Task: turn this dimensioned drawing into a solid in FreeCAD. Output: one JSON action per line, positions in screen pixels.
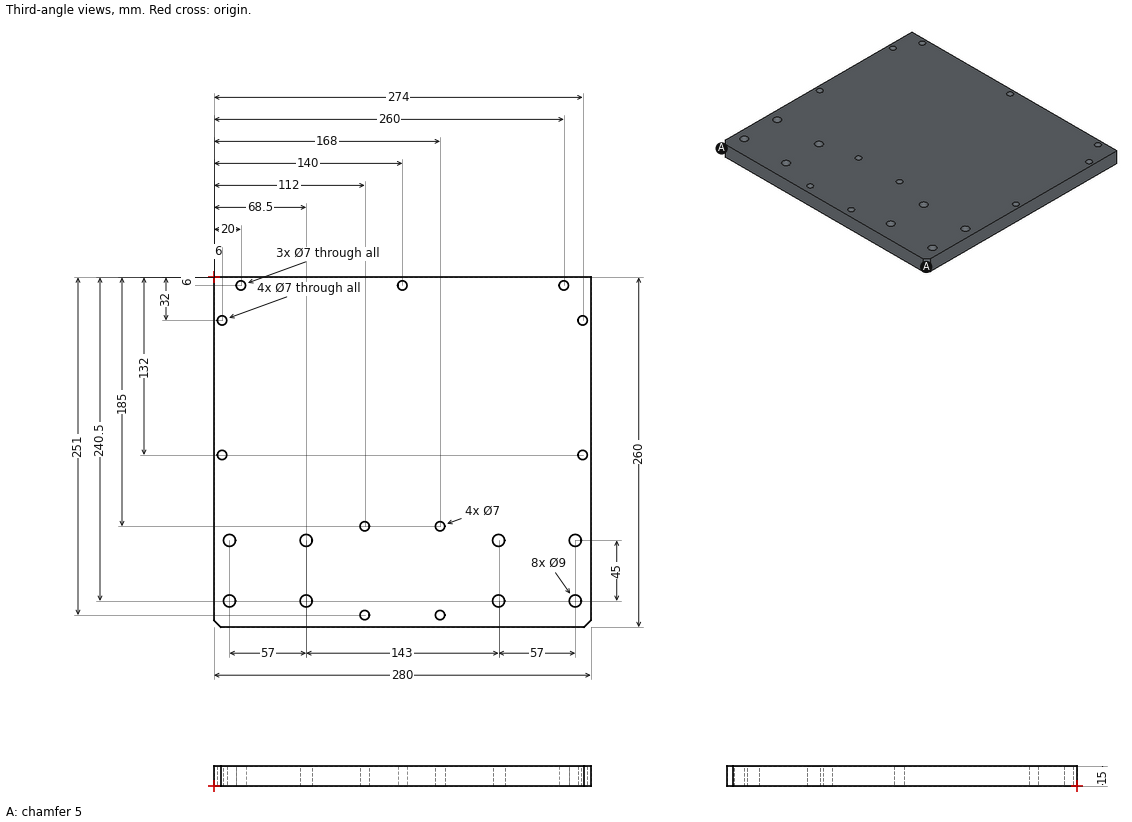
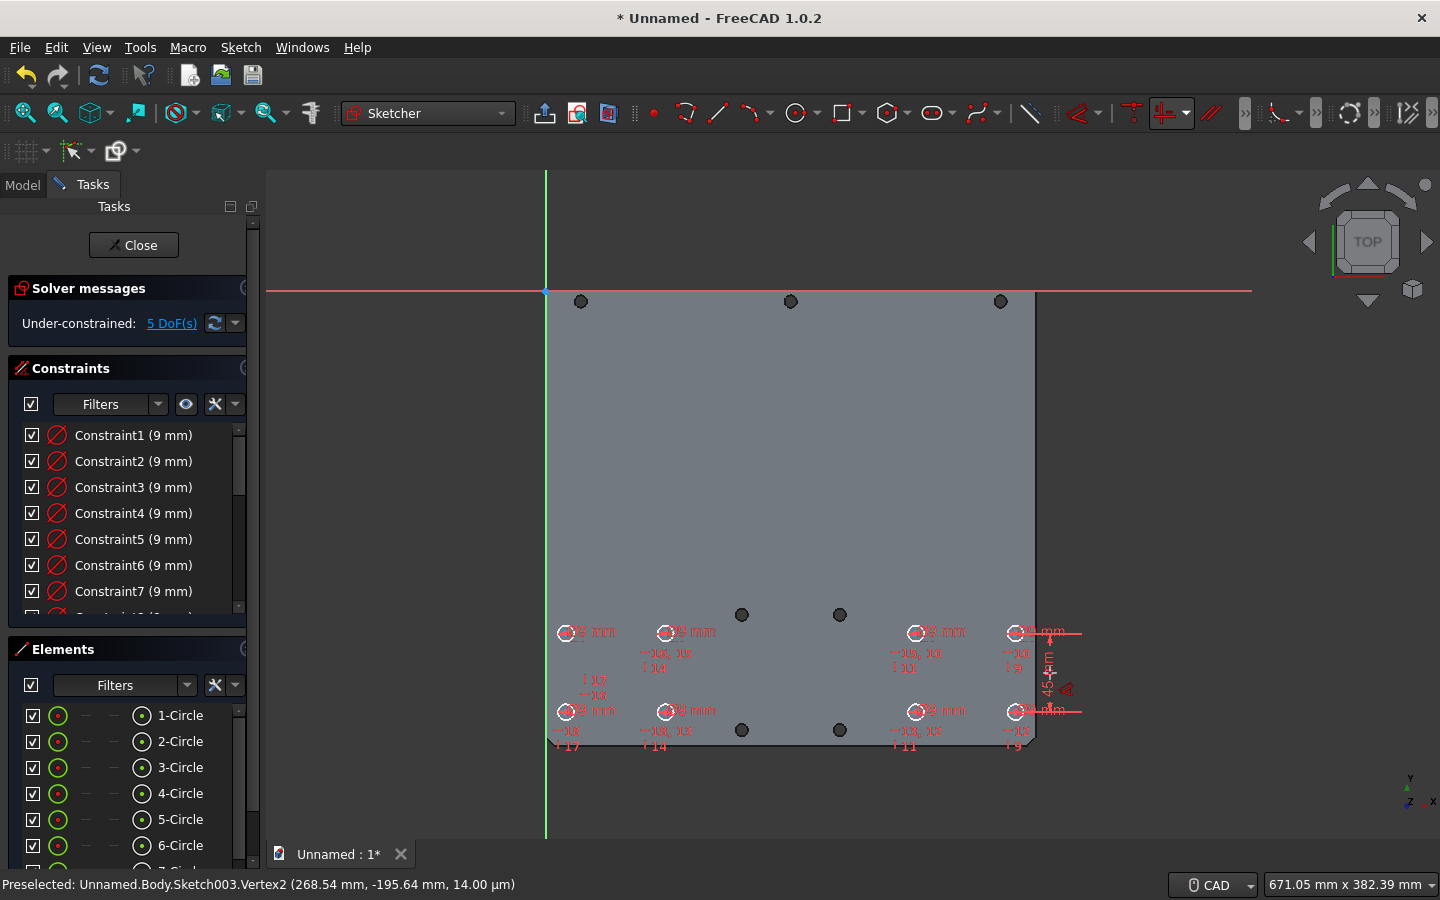
{"action": "left_click", "coordinate": [1016, 634]}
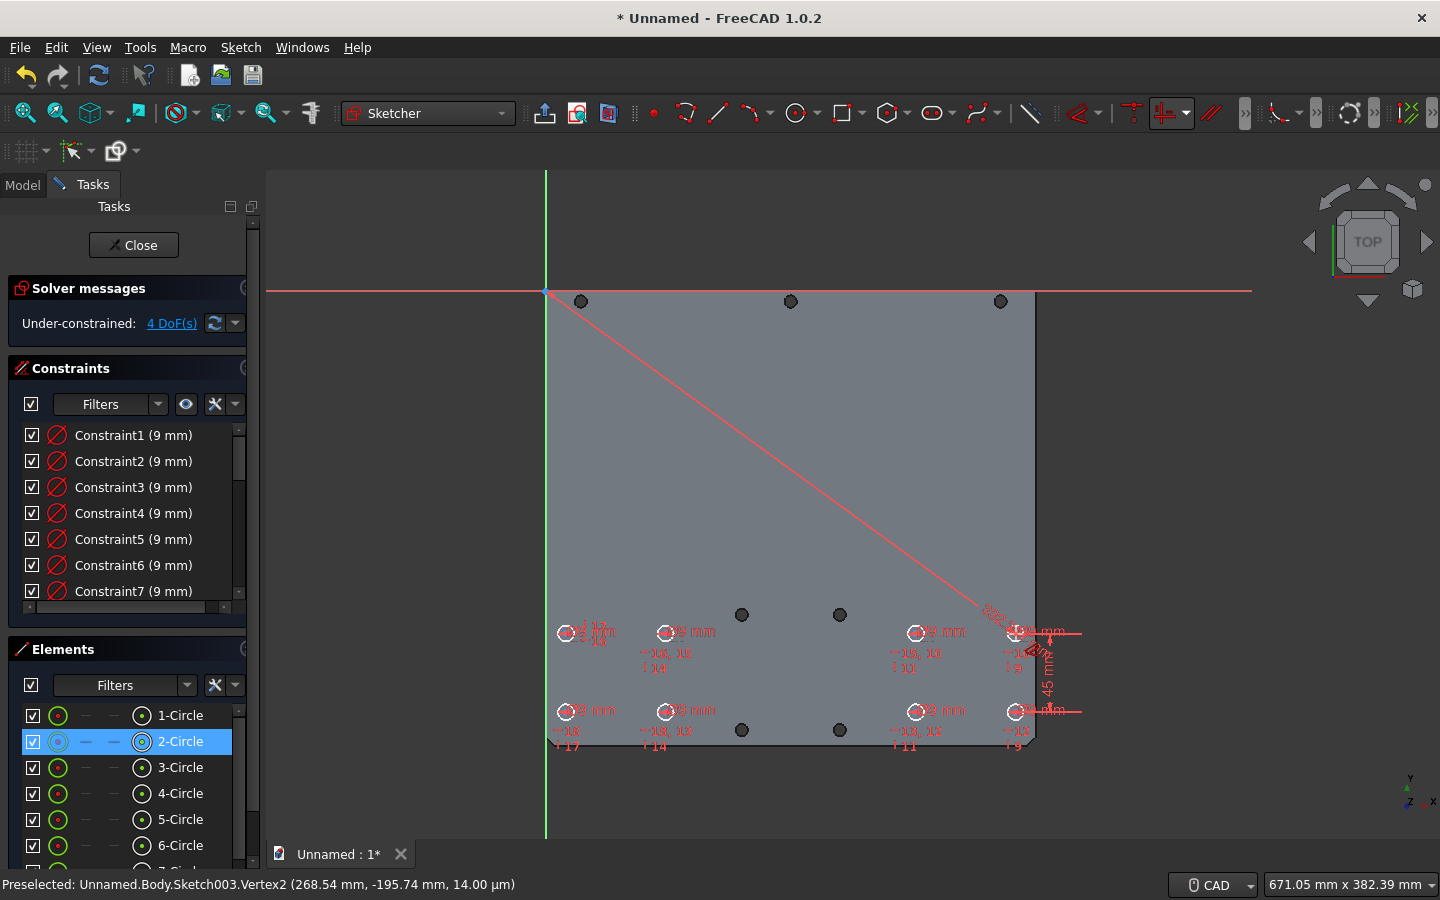
{"action": "left_click", "coordinate": [916, 634]}
{"action": "left_click", "coordinate": [966, 668]}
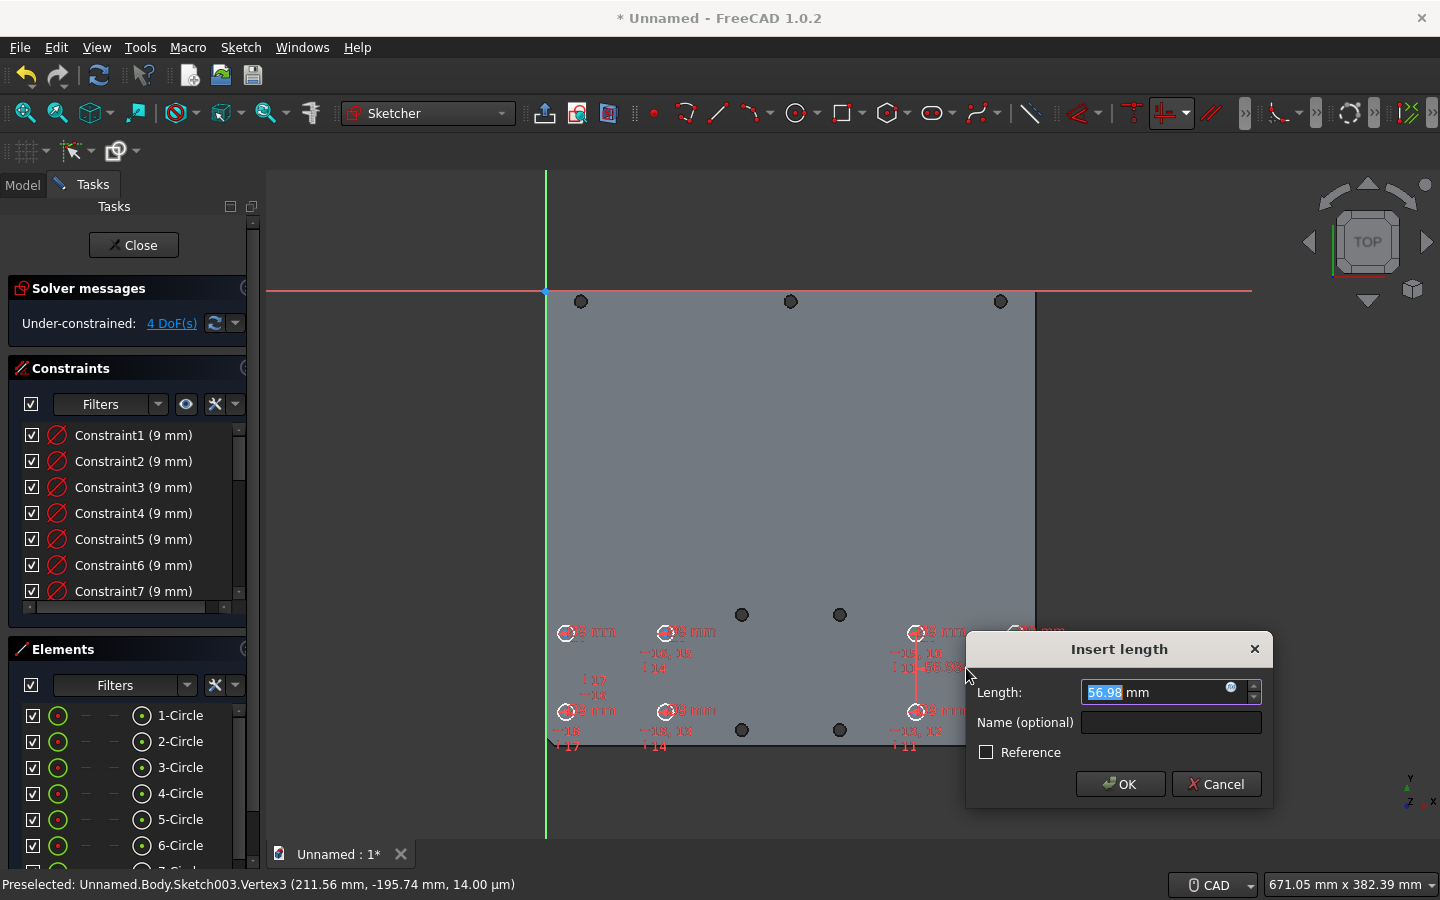
{"action": "type", "text": "57"}
{"action": "key", "text": "Return"}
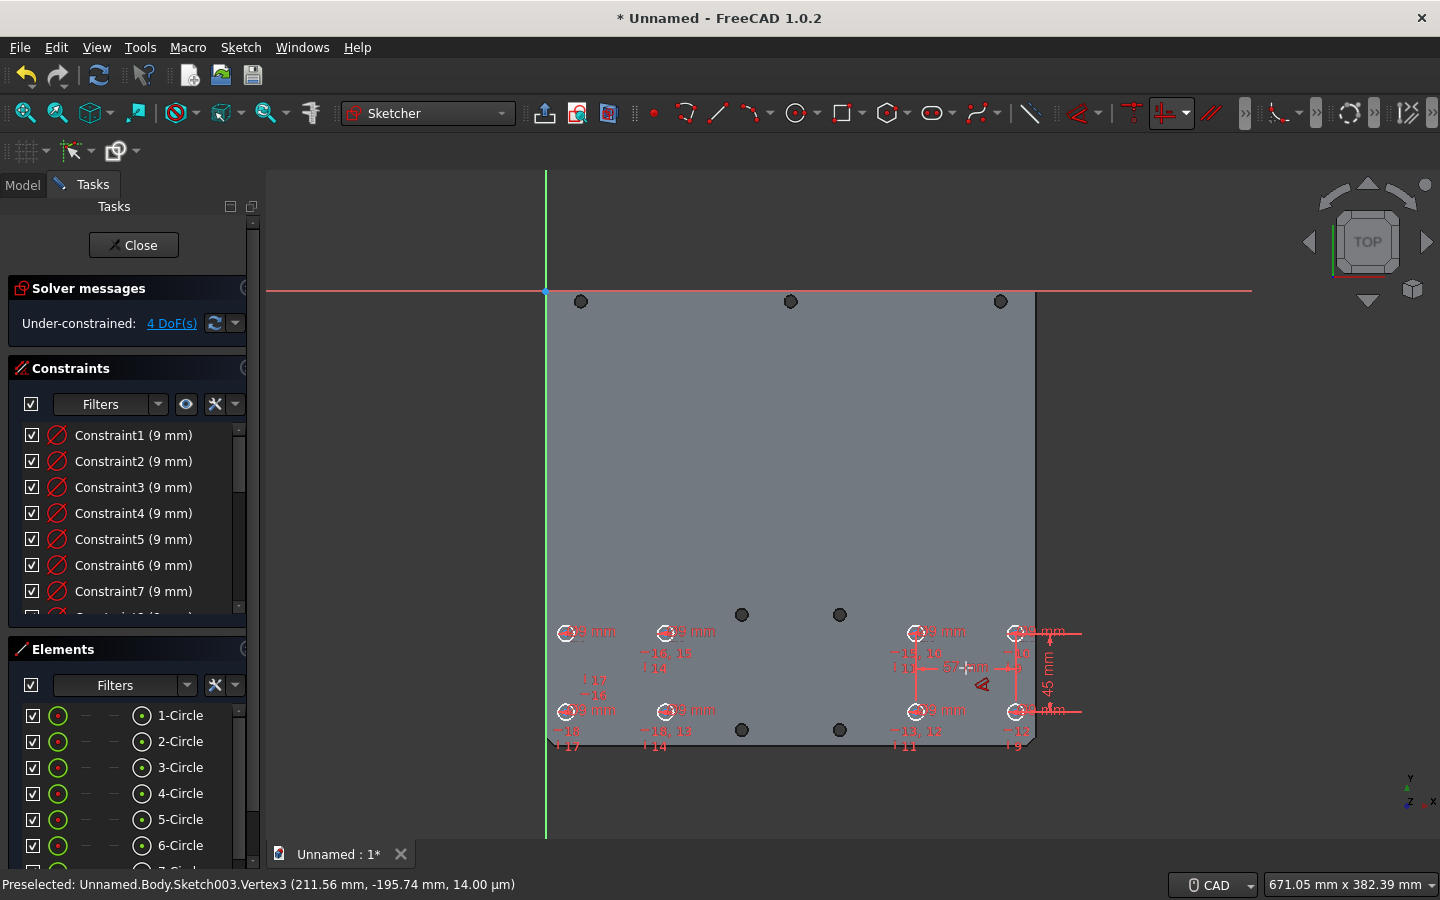
{"action": "left_click", "coordinate": [666, 634]}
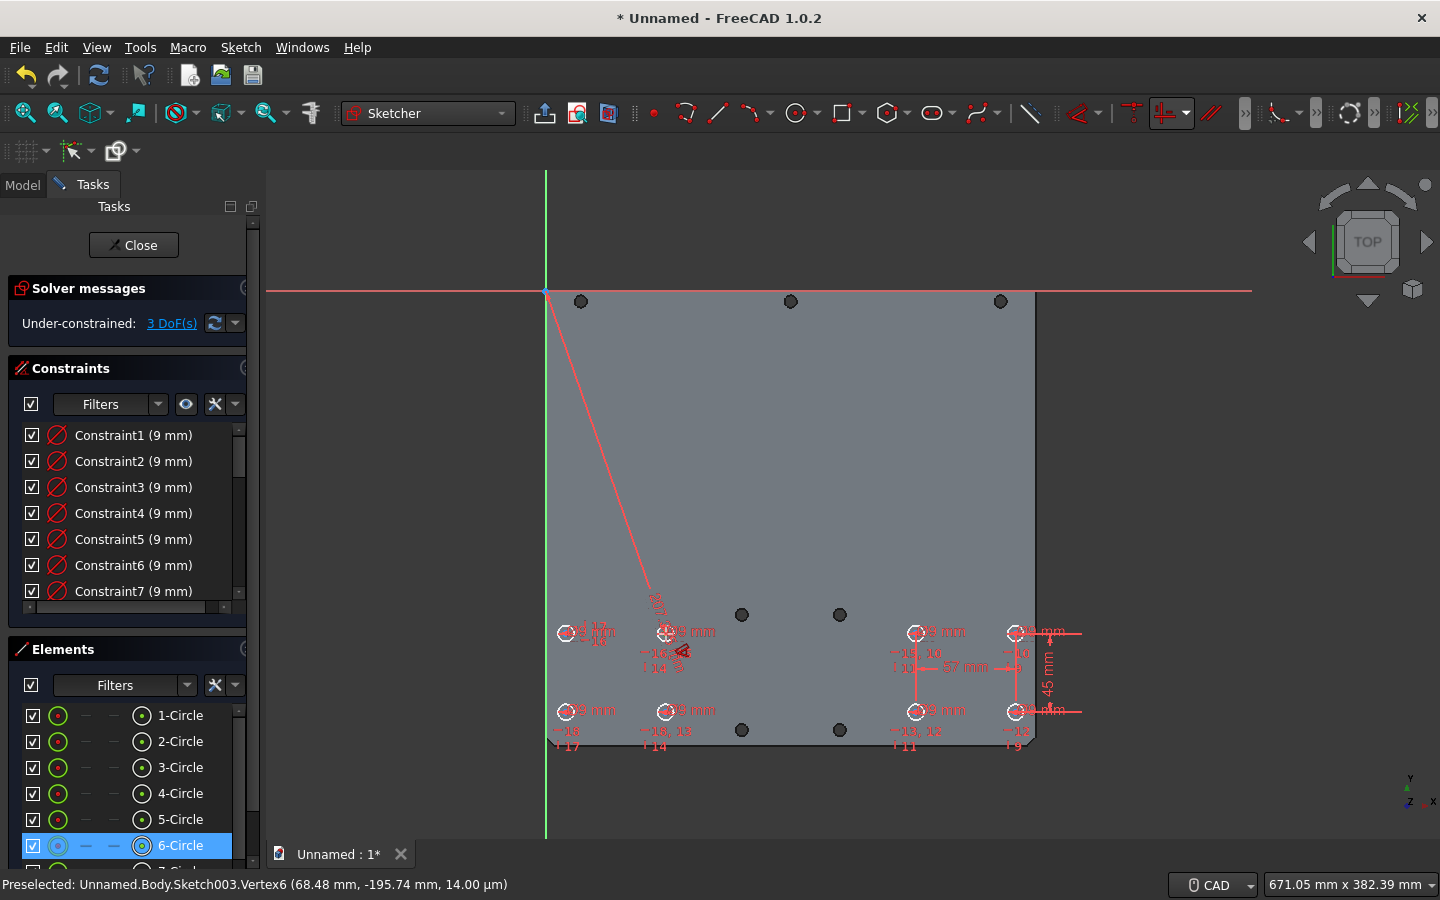
{"action": "left_click", "coordinate": [566, 634]}
{"action": "left_click", "coordinate": [616, 668]}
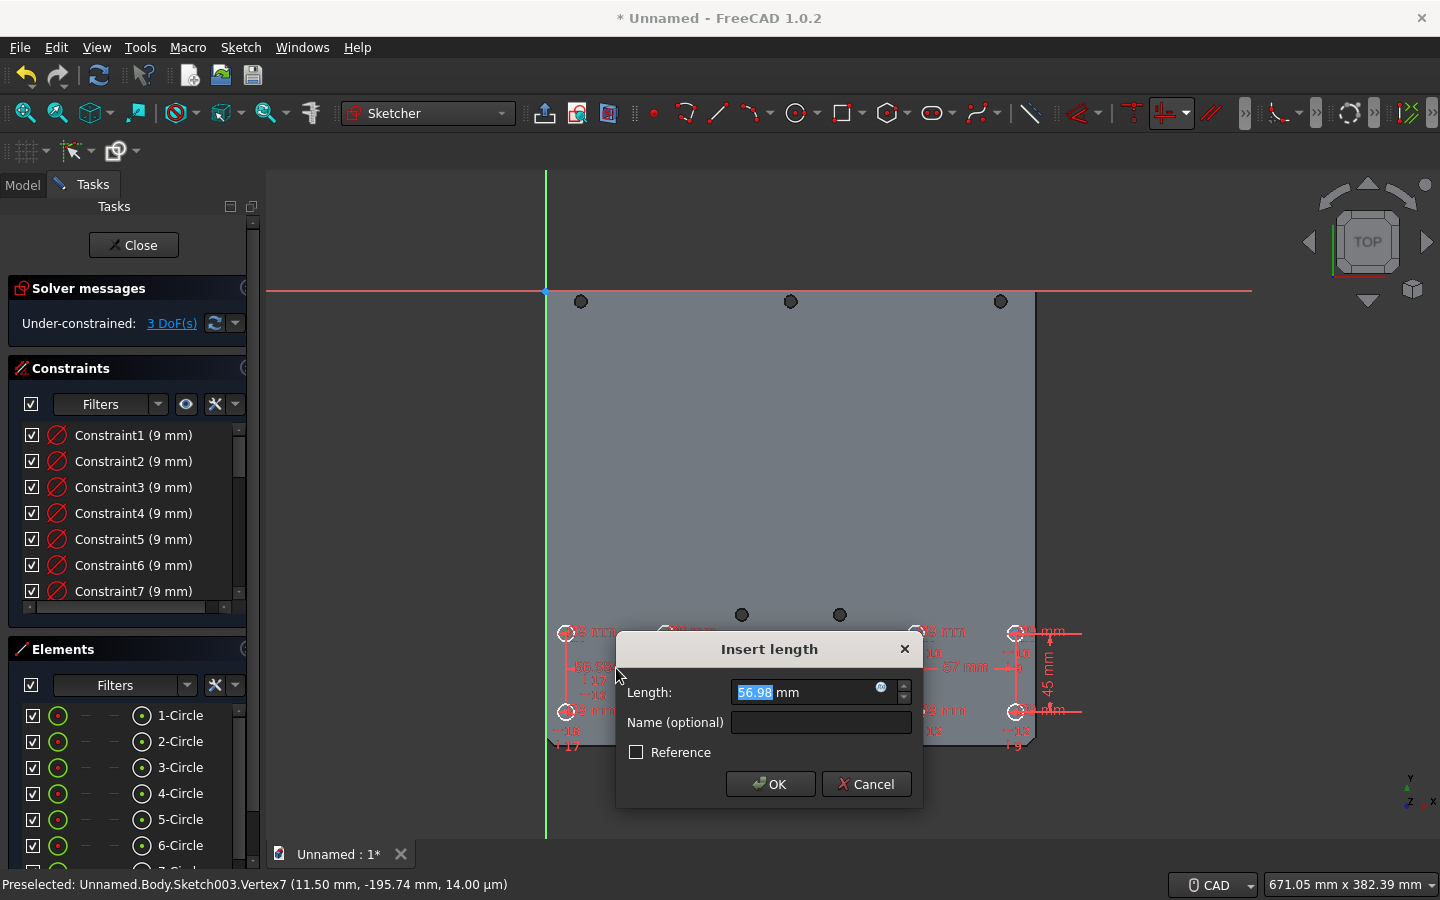
{"action": "type", "text": "57"}
{"action": "key", "text": "Return"}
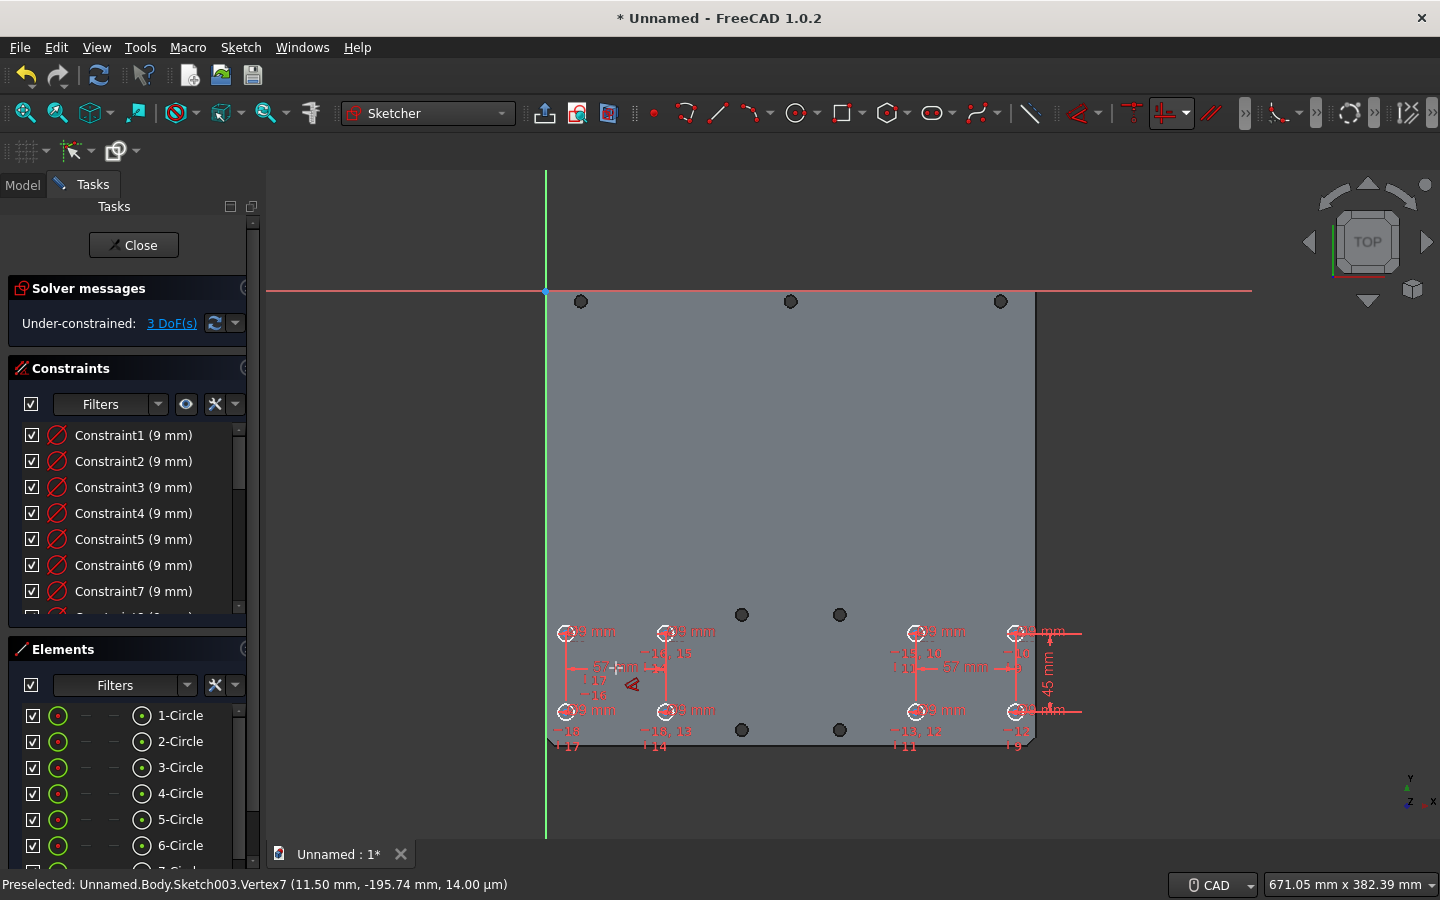
{"action": "left_click", "coordinate": [666, 712]}
{"action": "left_click", "coordinate": [606, 257]}